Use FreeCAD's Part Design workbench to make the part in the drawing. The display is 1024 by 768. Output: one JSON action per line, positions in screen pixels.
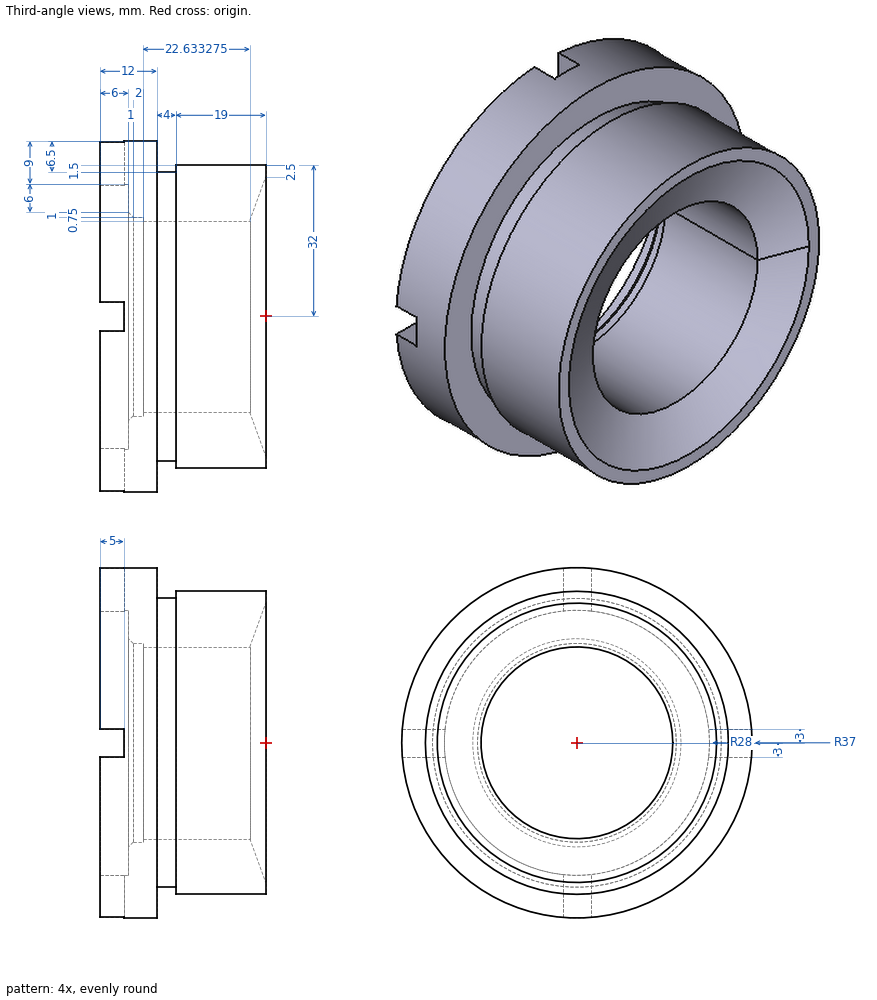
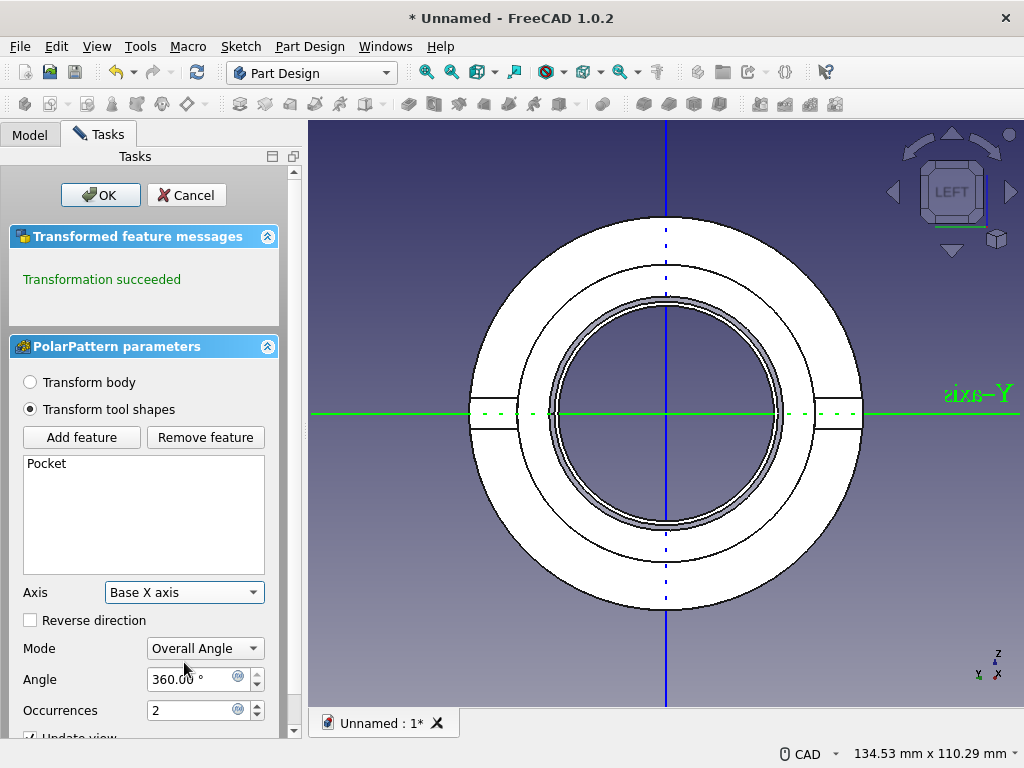
{"action": "triple_click", "coordinate": [199, 710]}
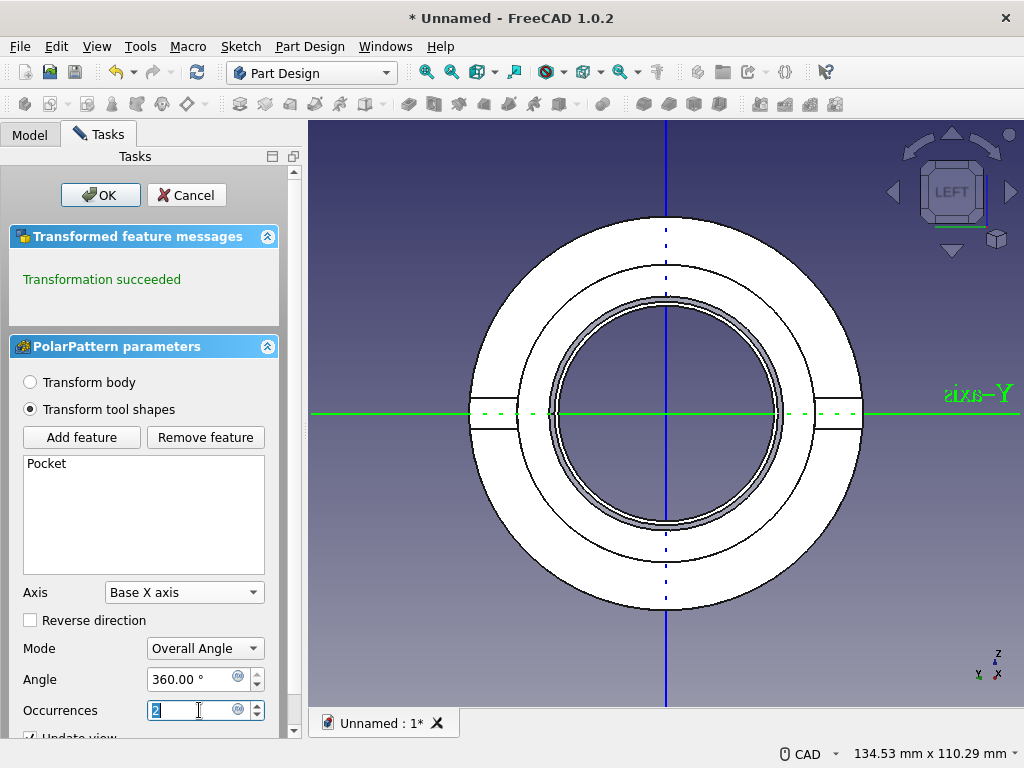
{"action": "type", "text": "4"}
{"action": "key", "text": "Tab"}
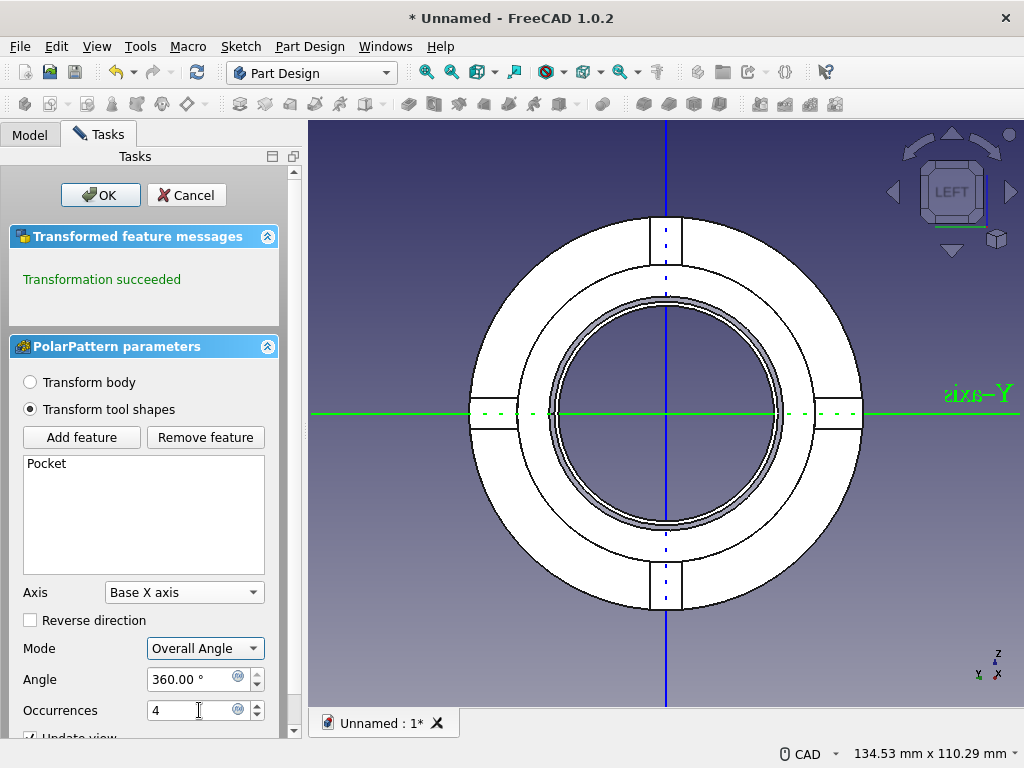
{"action": "left_click", "coordinate": [101, 195]}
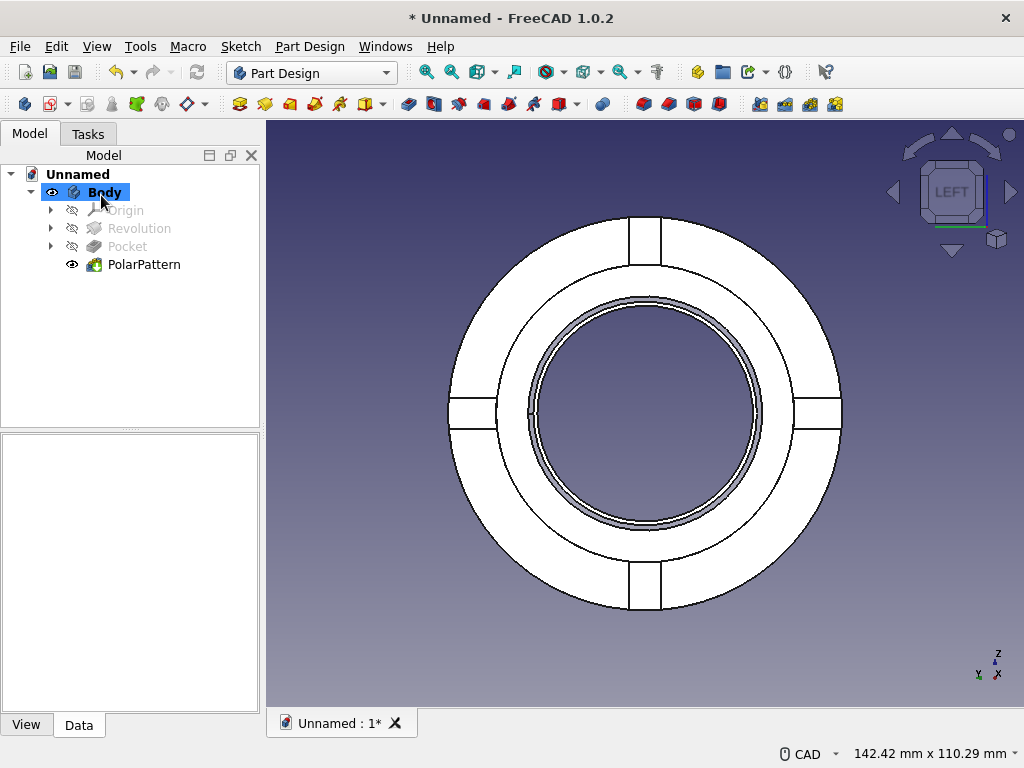
{"action": "key", "text": "0"}